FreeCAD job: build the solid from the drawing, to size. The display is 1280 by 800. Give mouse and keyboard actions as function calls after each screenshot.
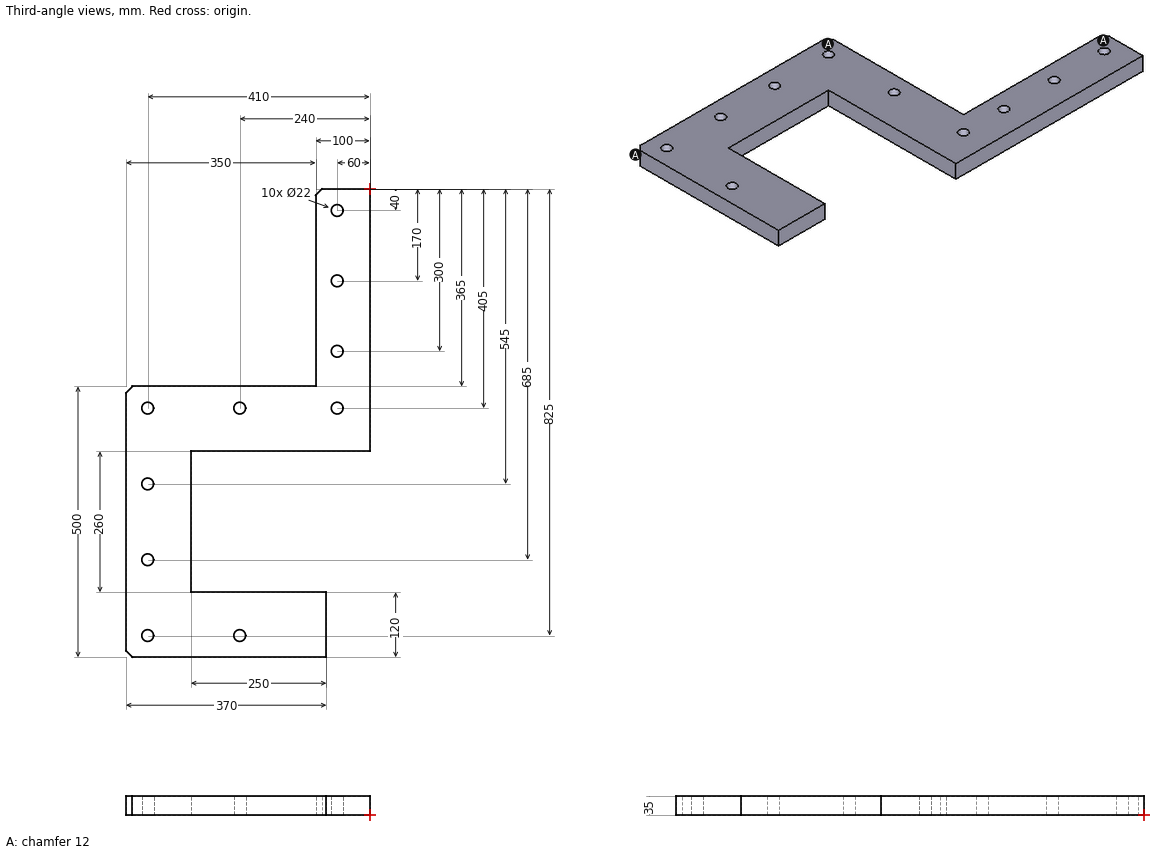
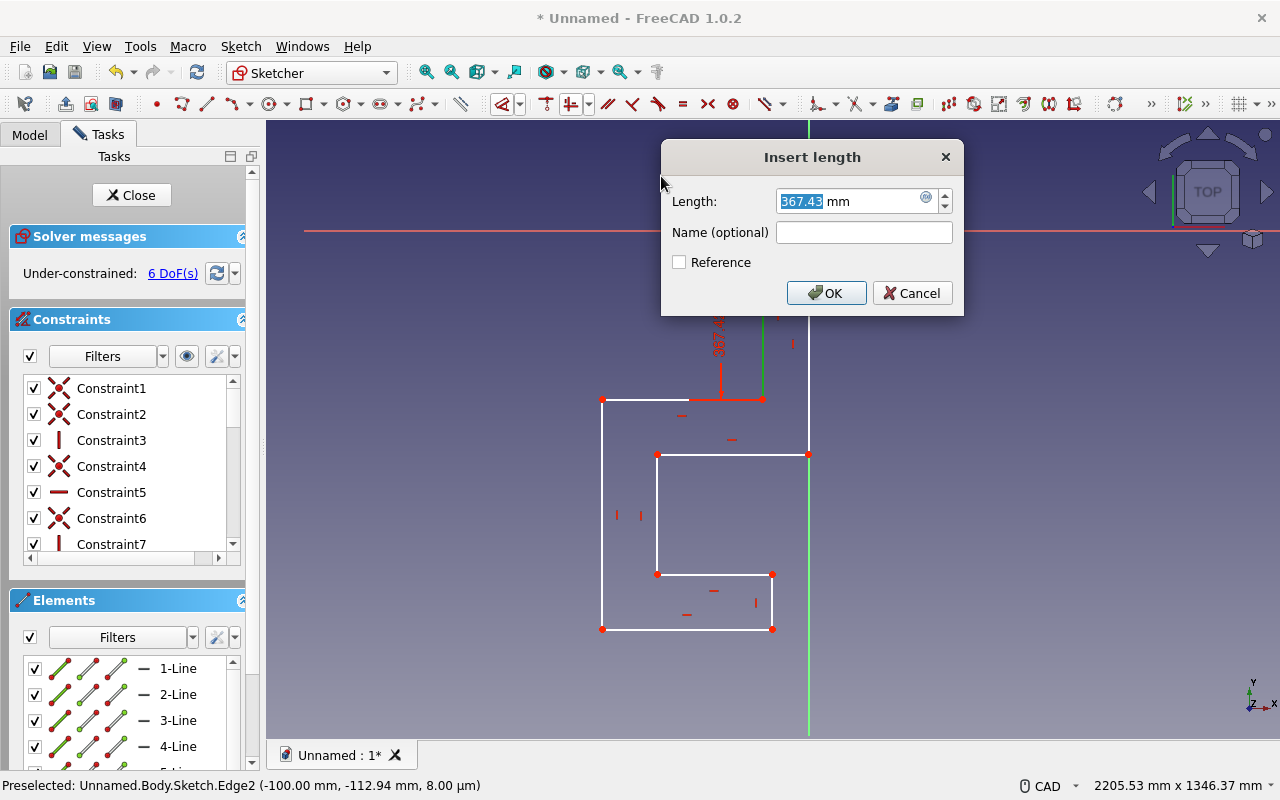
text(365)
key(Return)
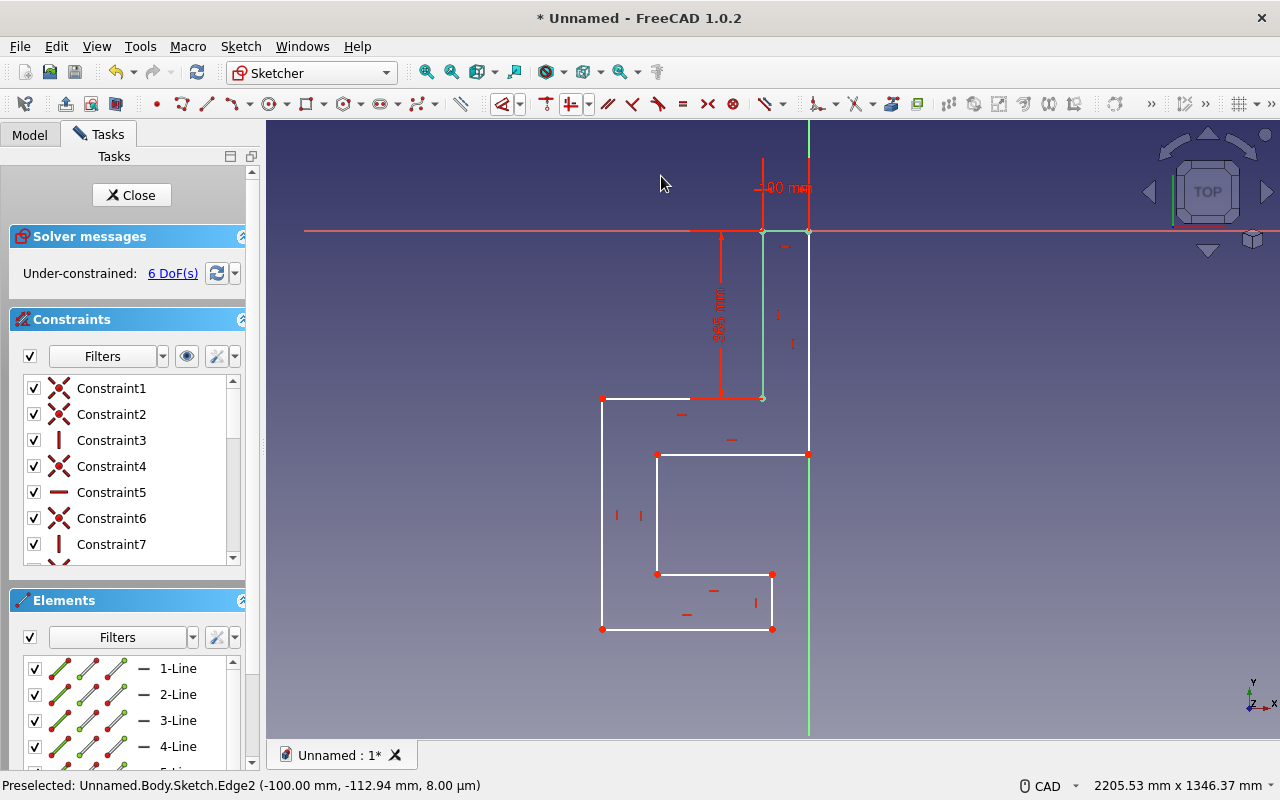
click(714, 399)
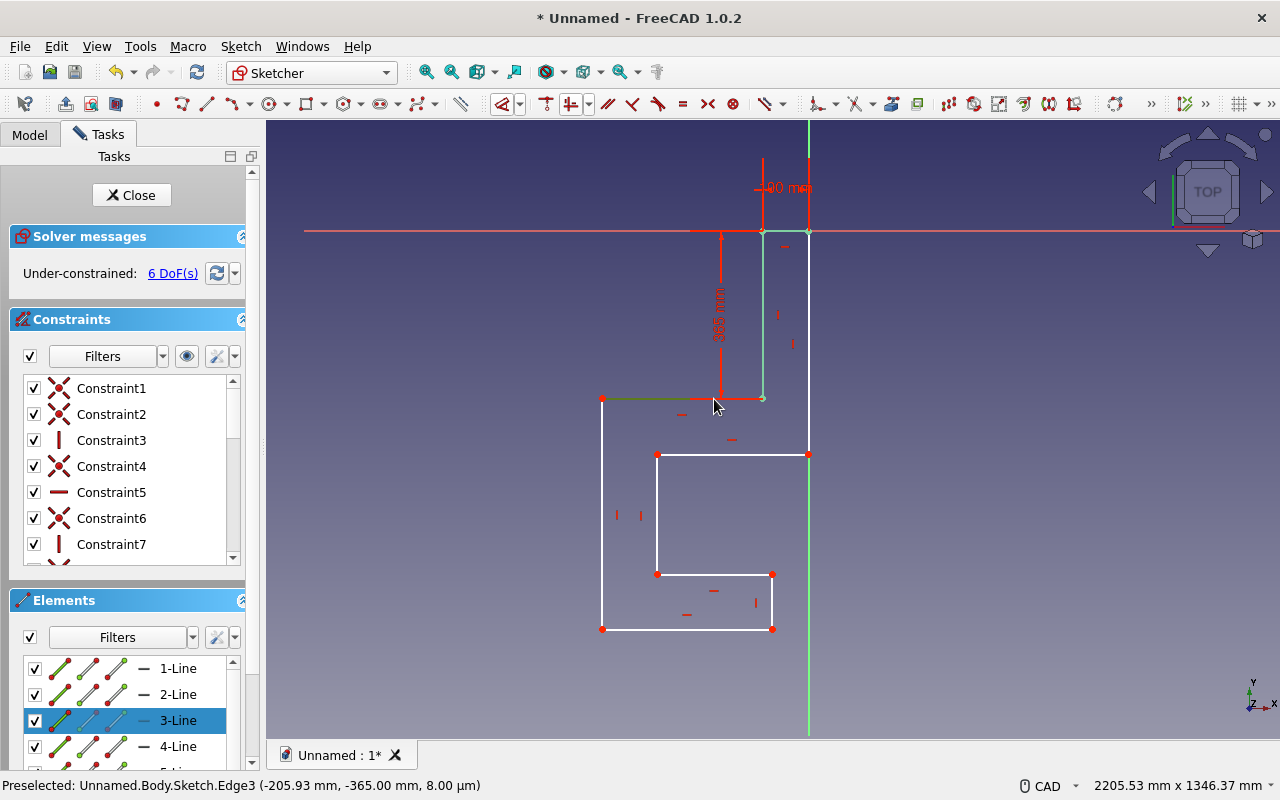
click(520, 104)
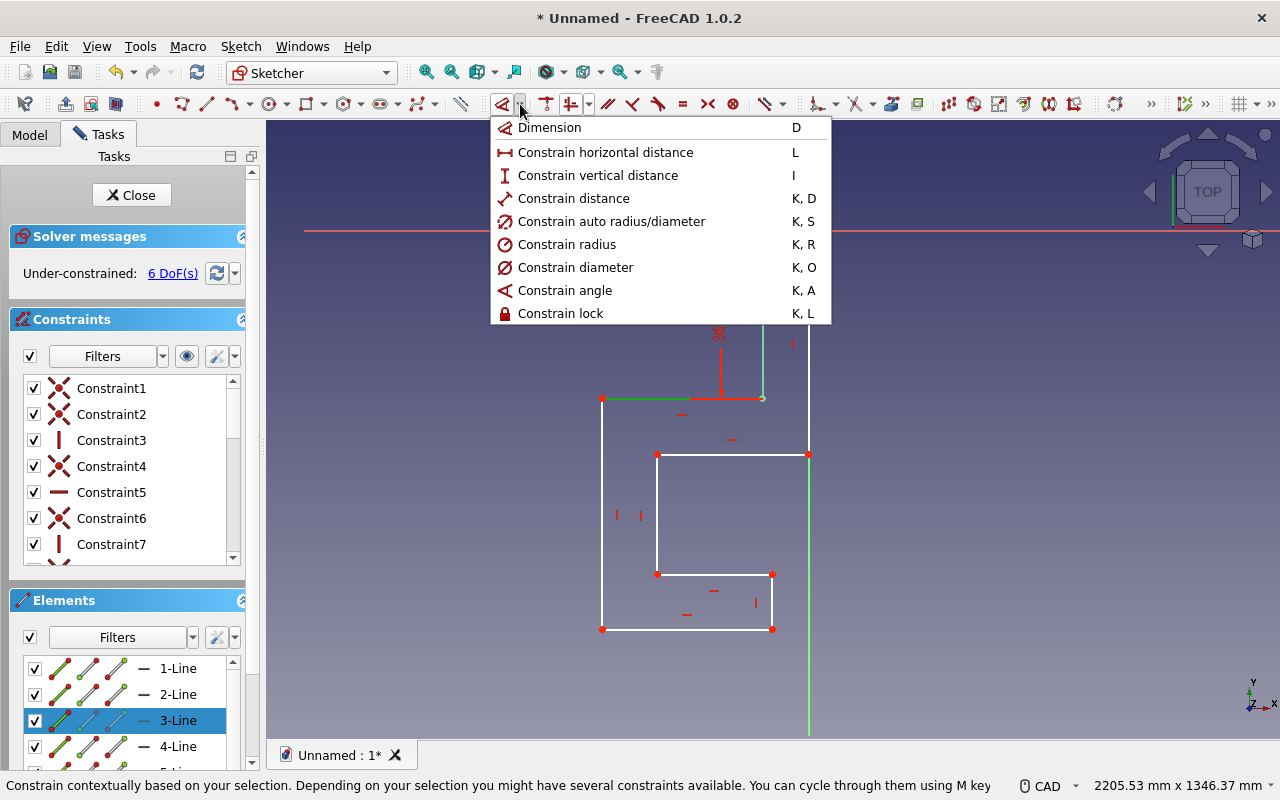
click(661, 152)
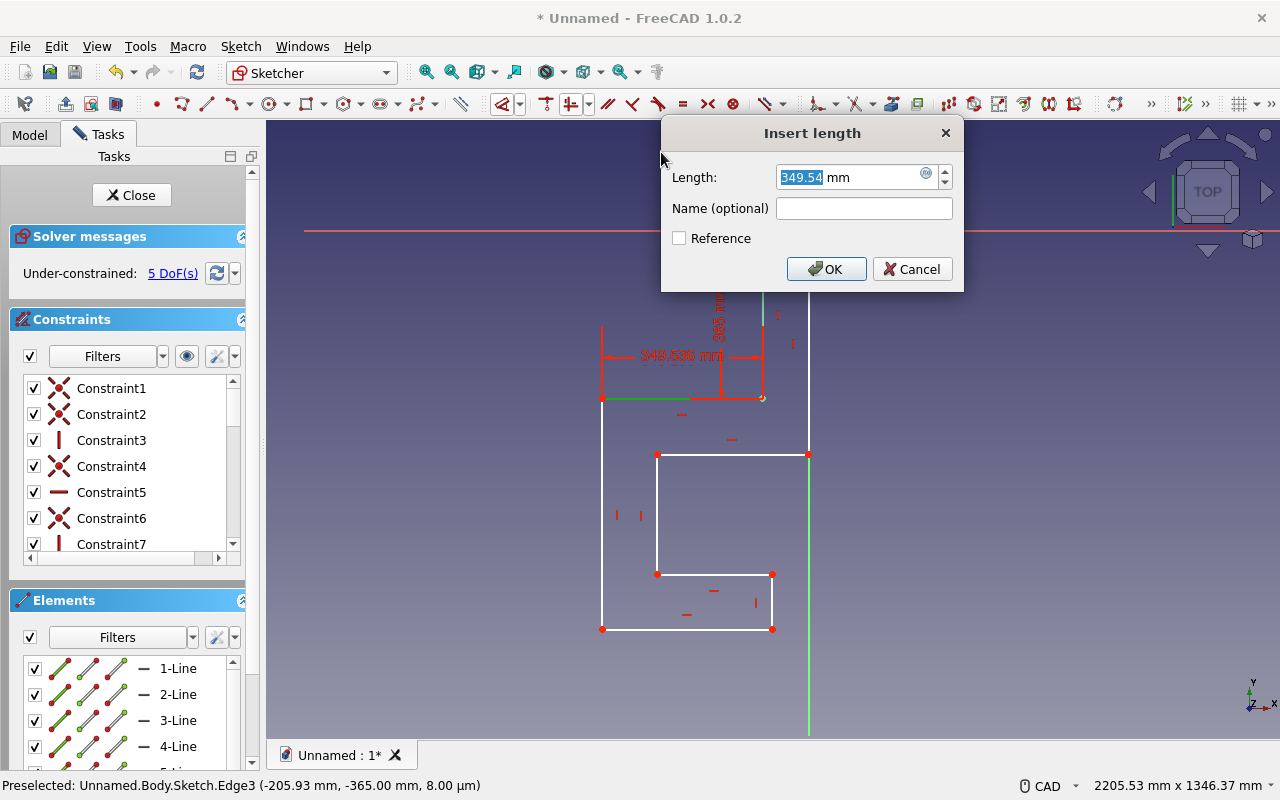
text(350)
key(Return)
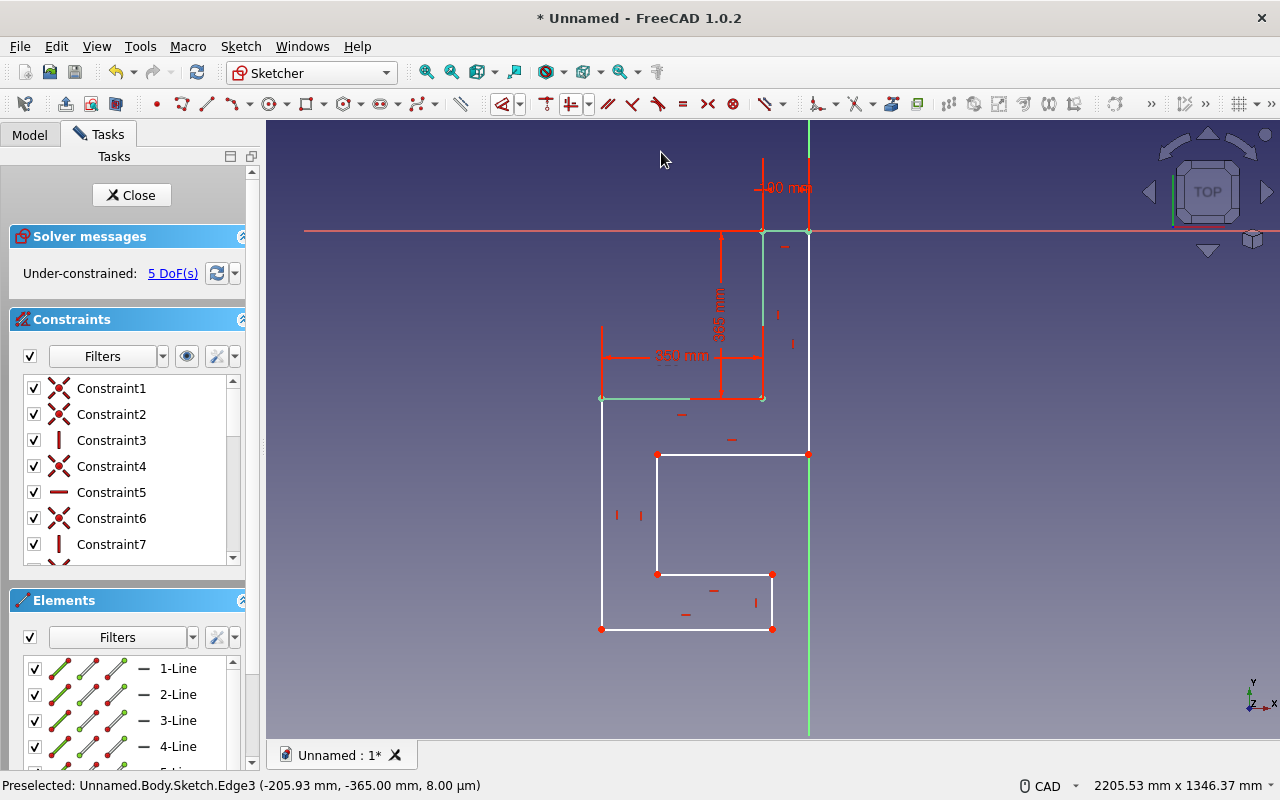
click(602, 468)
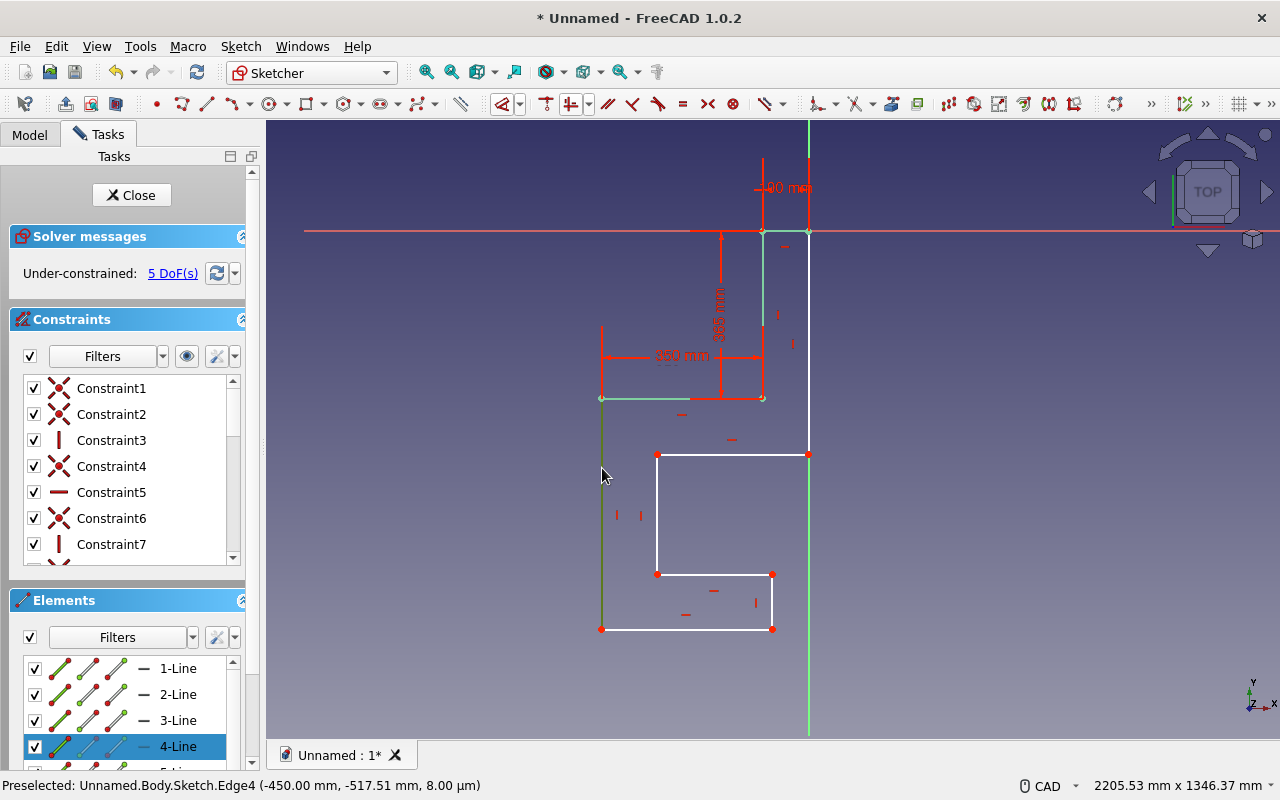
click(520, 104)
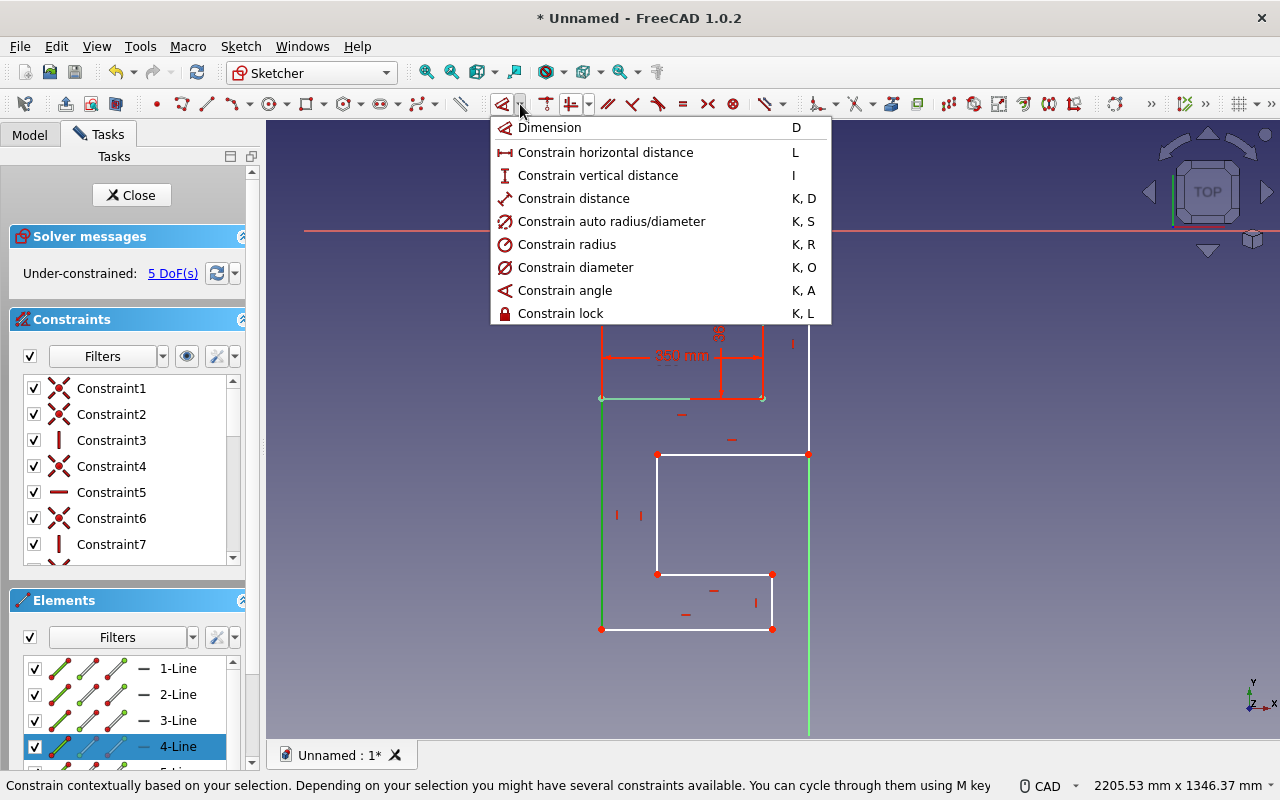
click(661, 176)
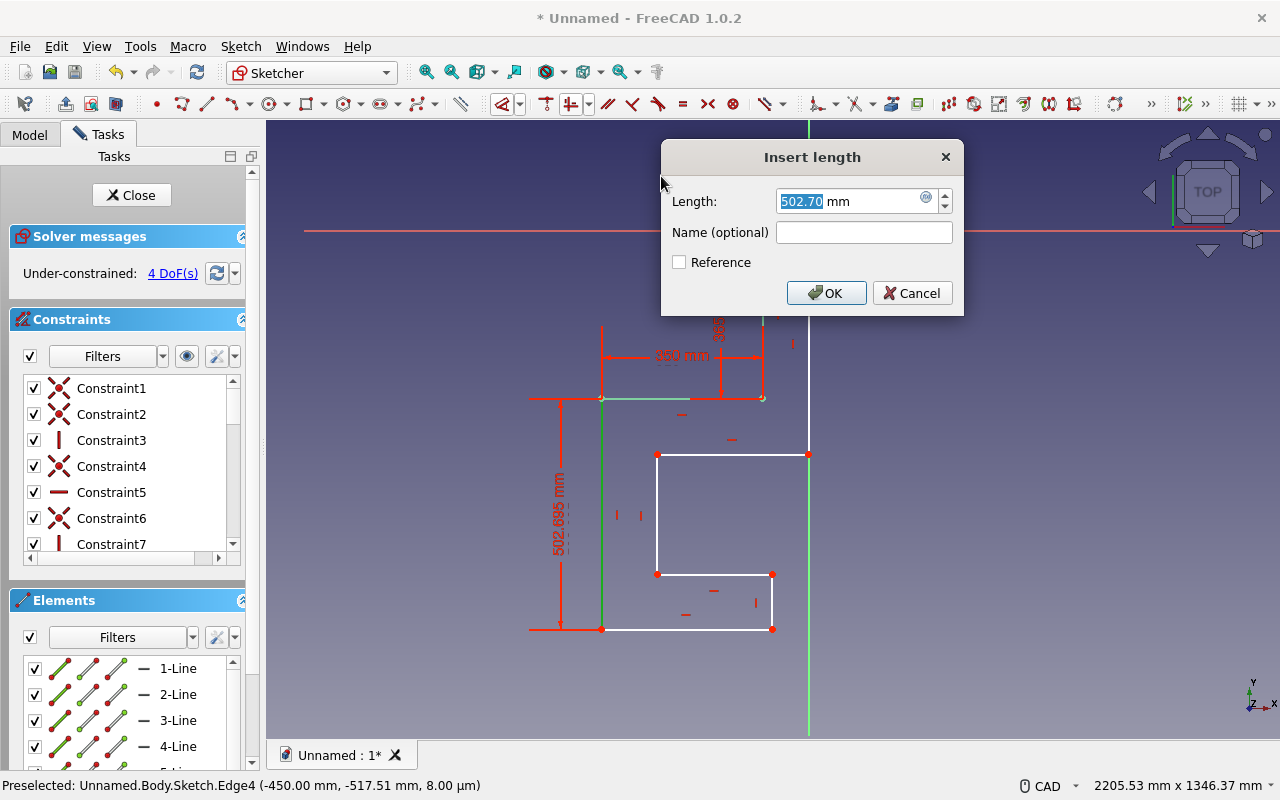
text(500)
key(Return)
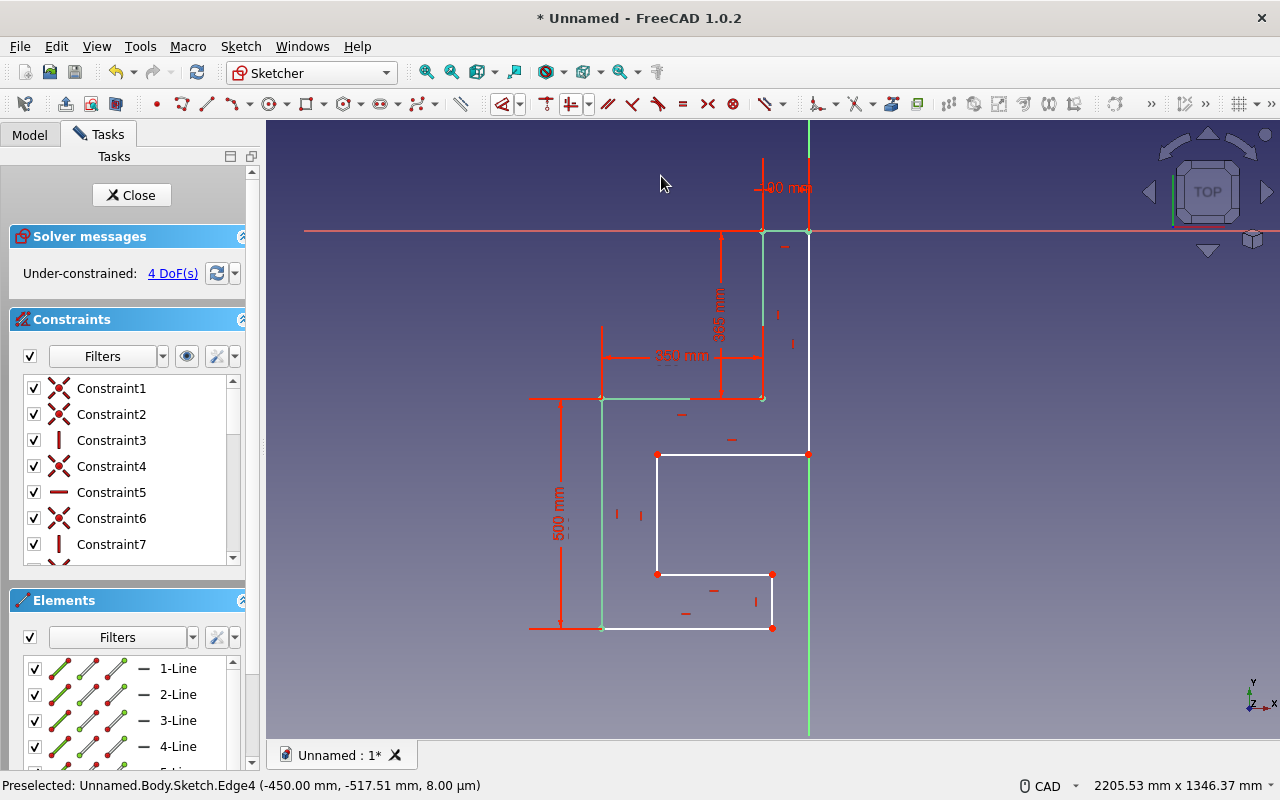
click(653, 629)